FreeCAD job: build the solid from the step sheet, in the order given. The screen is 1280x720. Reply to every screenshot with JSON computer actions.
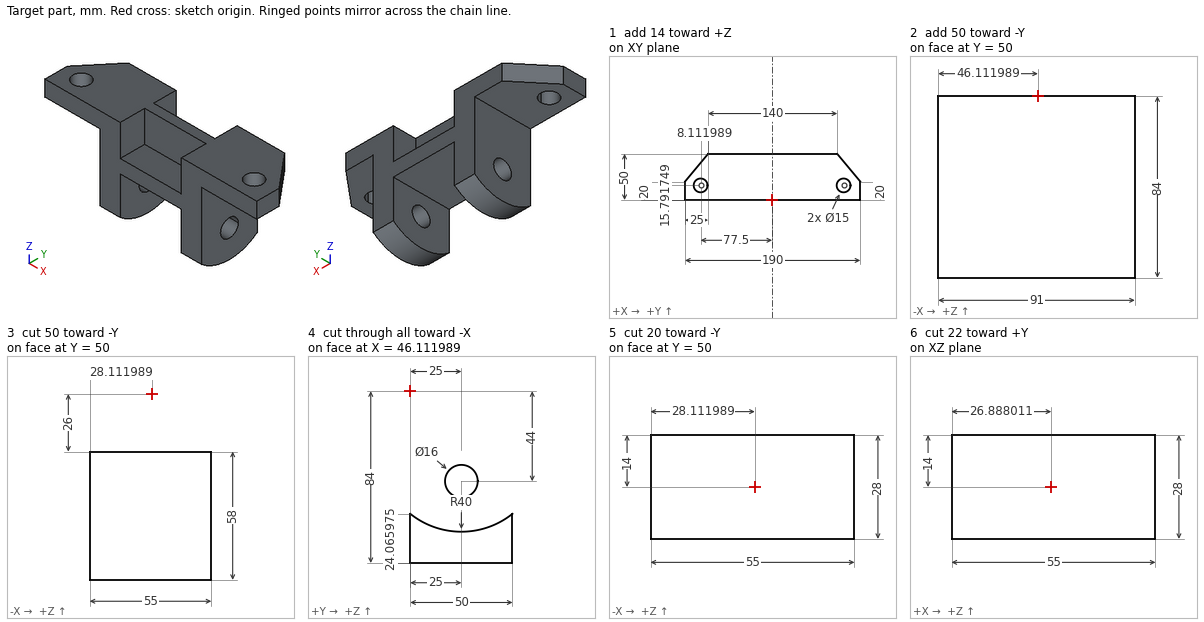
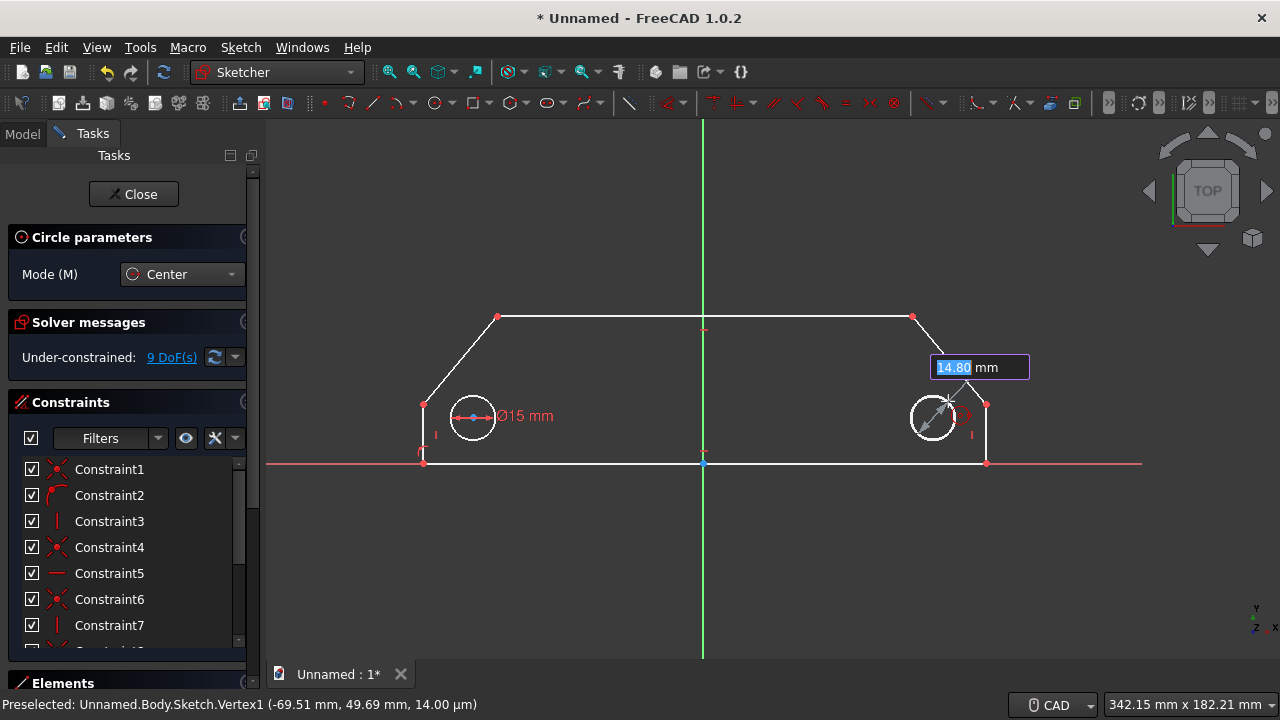
{"action": "type", "text": "15"}
{"action": "key", "text": "Return"}
{"action": "key", "text": "Escape"}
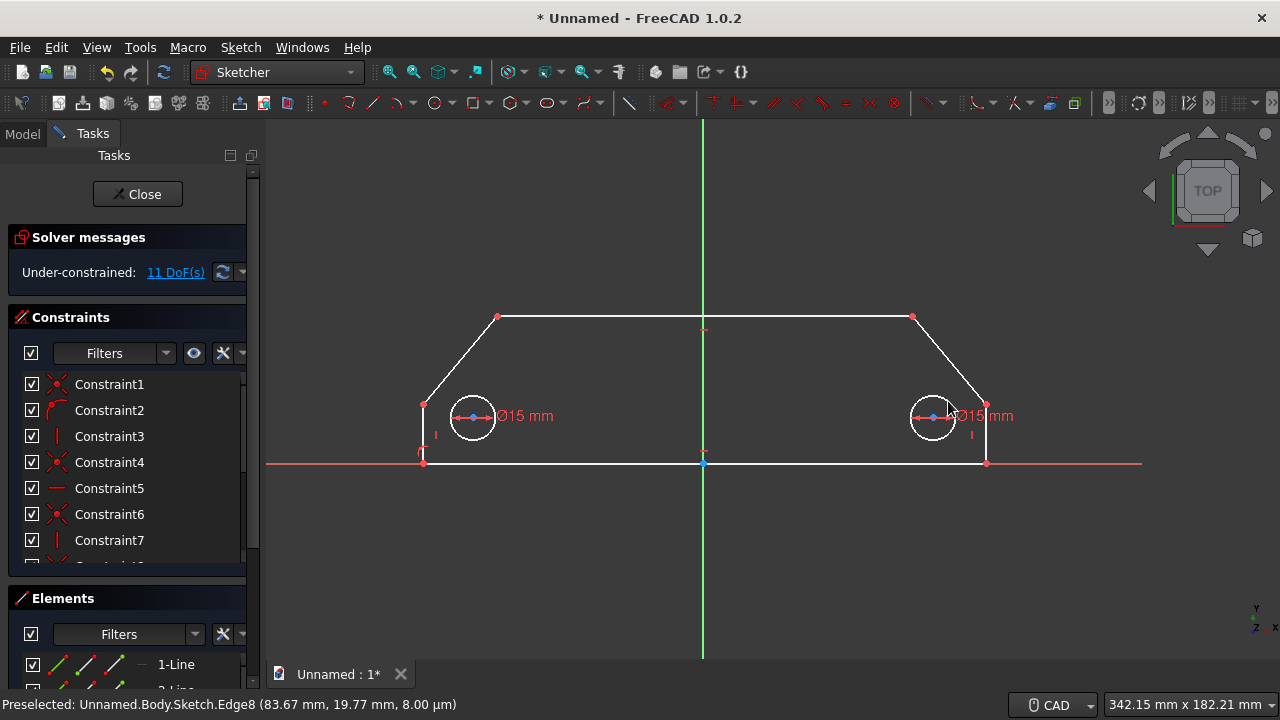
{"action": "left_click", "coordinate": [473, 418]}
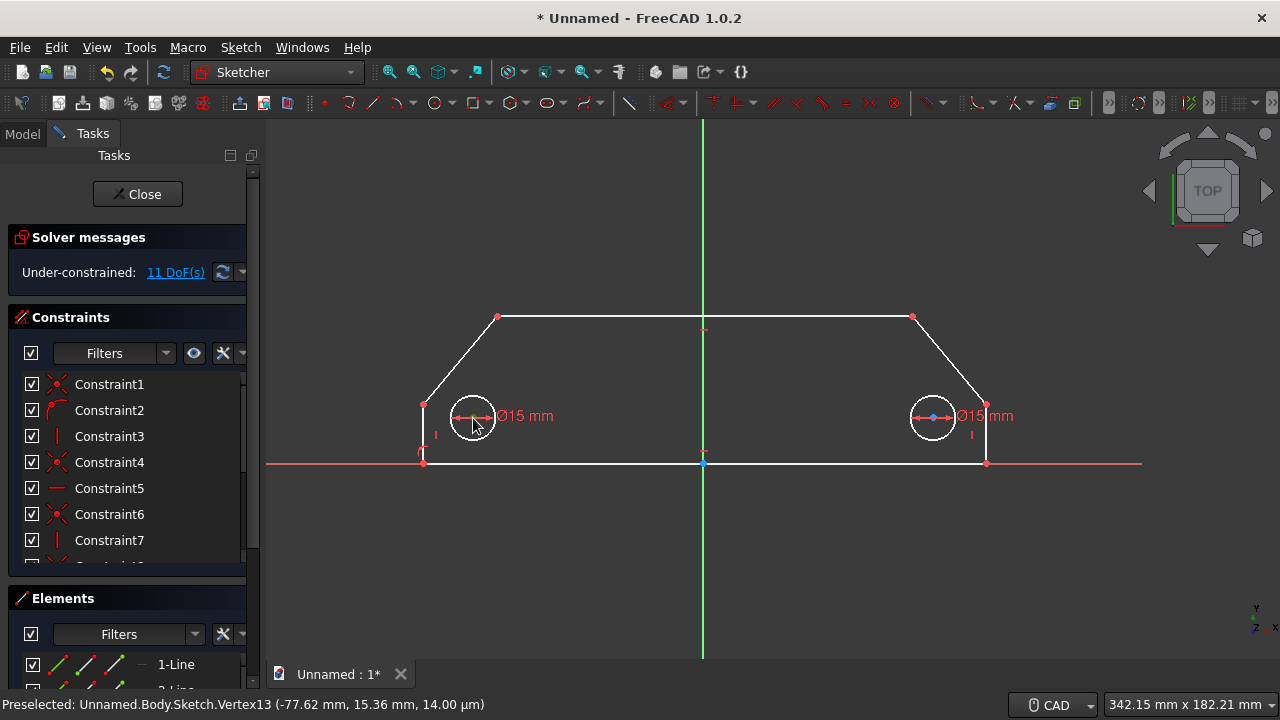
{"action": "left_click", "coordinate": [933, 418]}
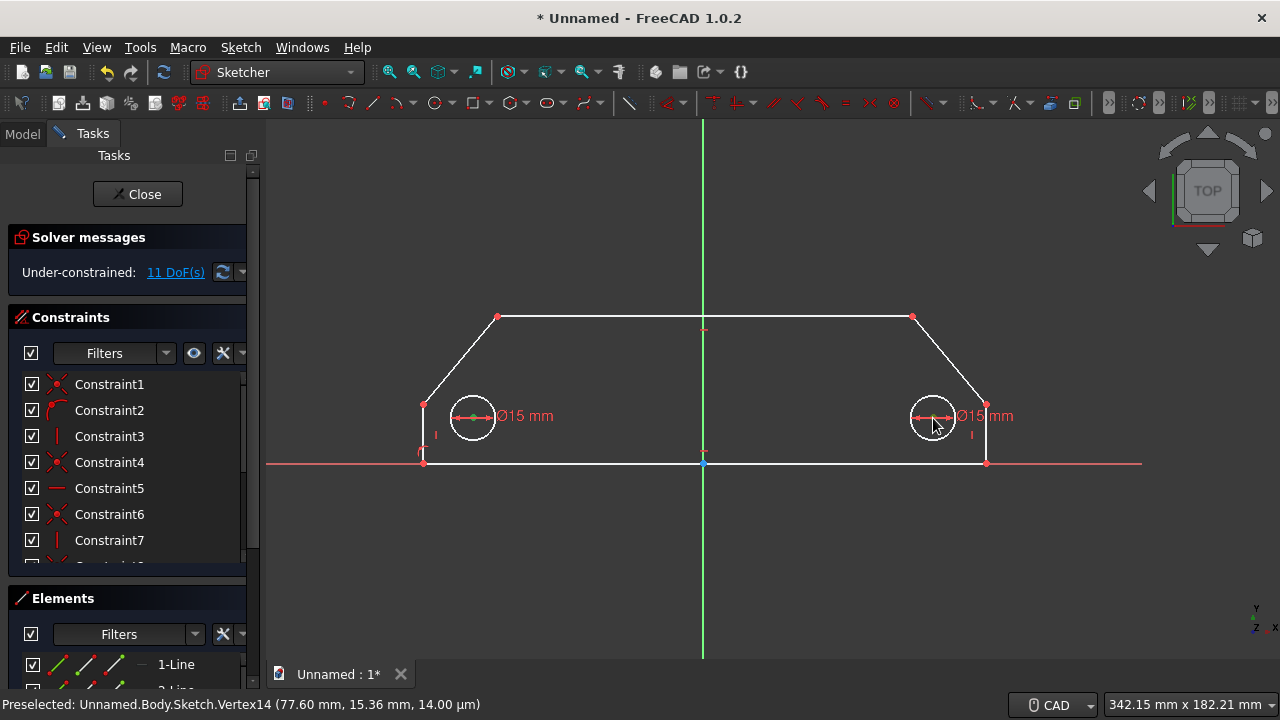
{"action": "left_click", "coordinate": [703, 596]}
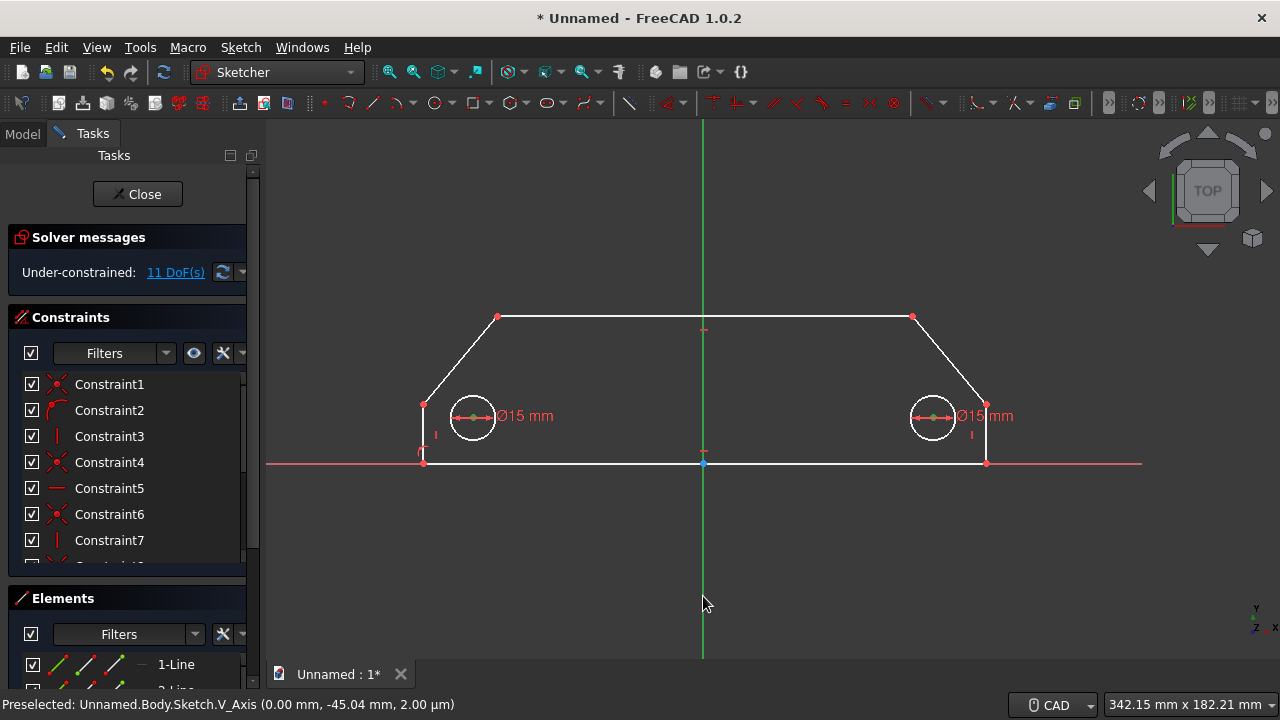
{"action": "left_click", "coordinate": [870, 104]}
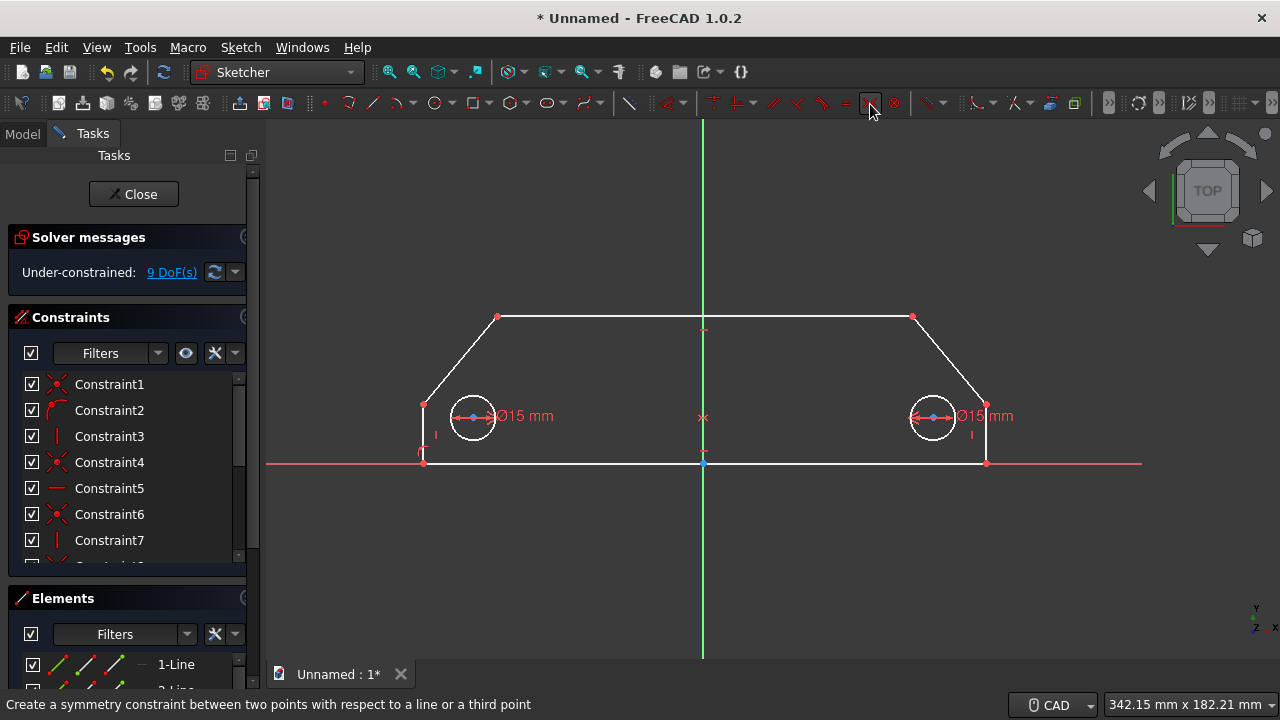
{"action": "left_click", "coordinate": [668, 104]}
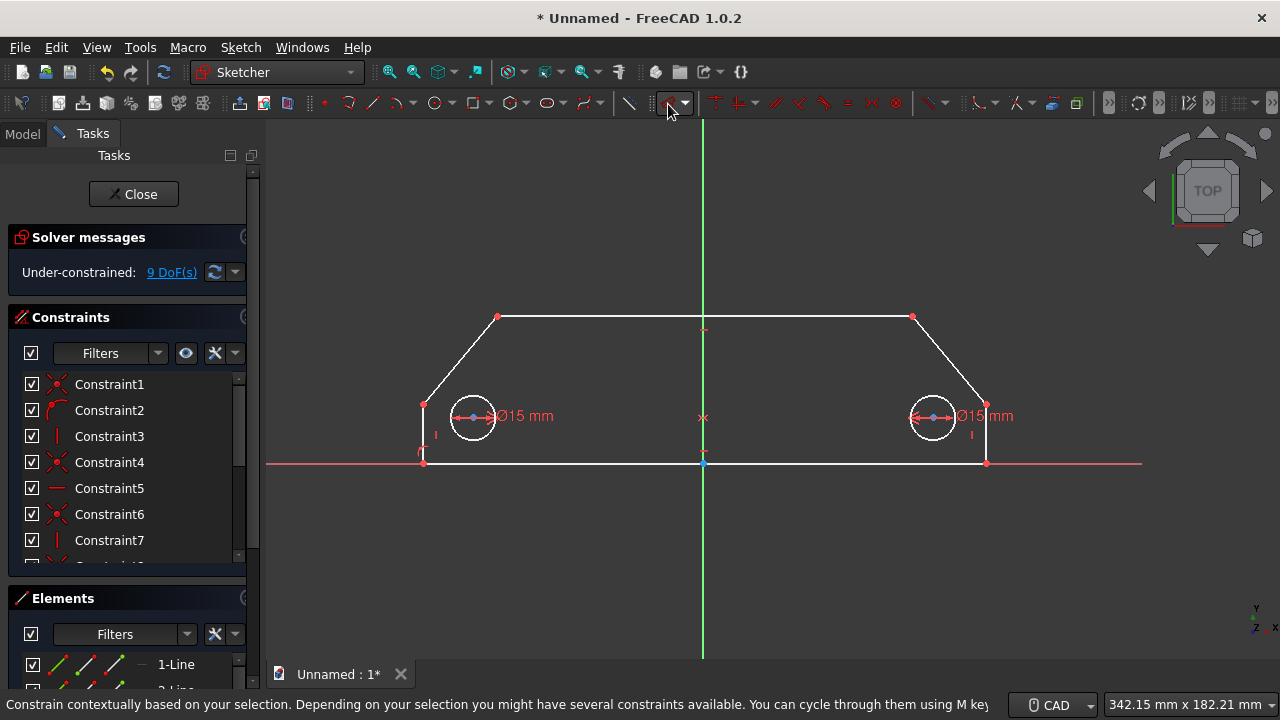
{"action": "left_click", "coordinate": [423, 423]}
{"action": "left_click", "coordinate": [389, 434]}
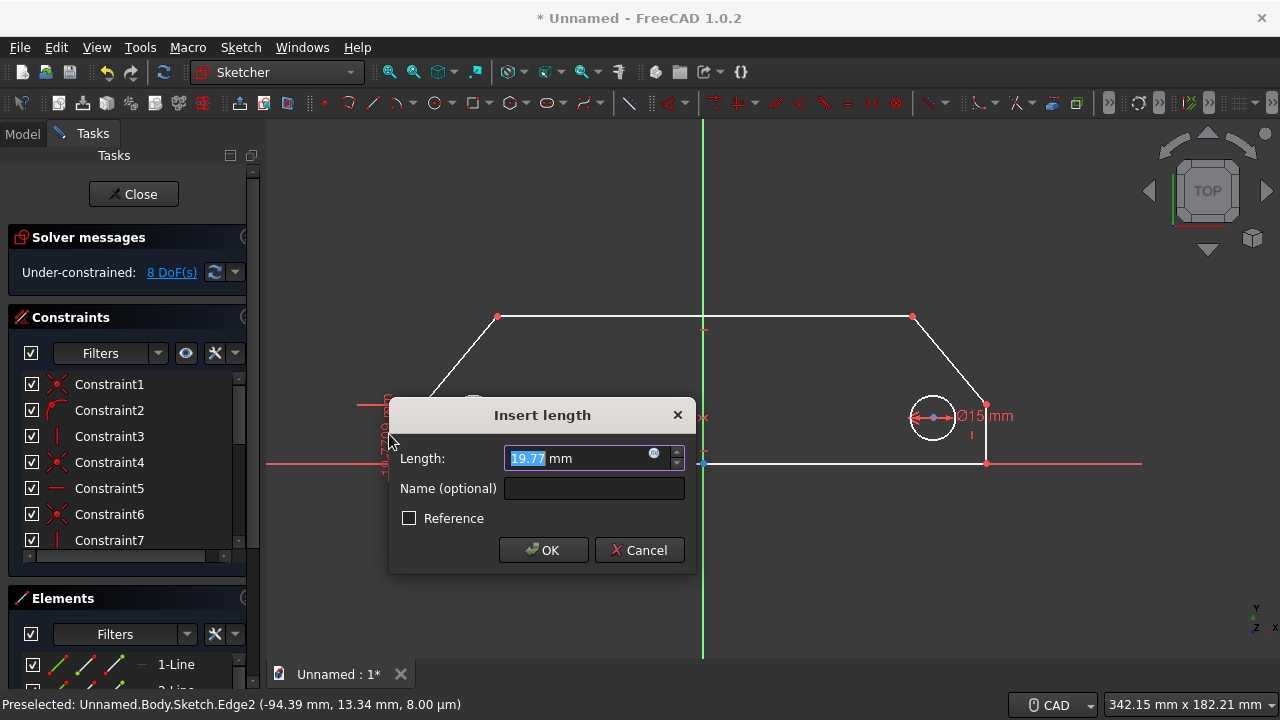
{"action": "type", "text": "20"}
{"action": "key", "text": "Return"}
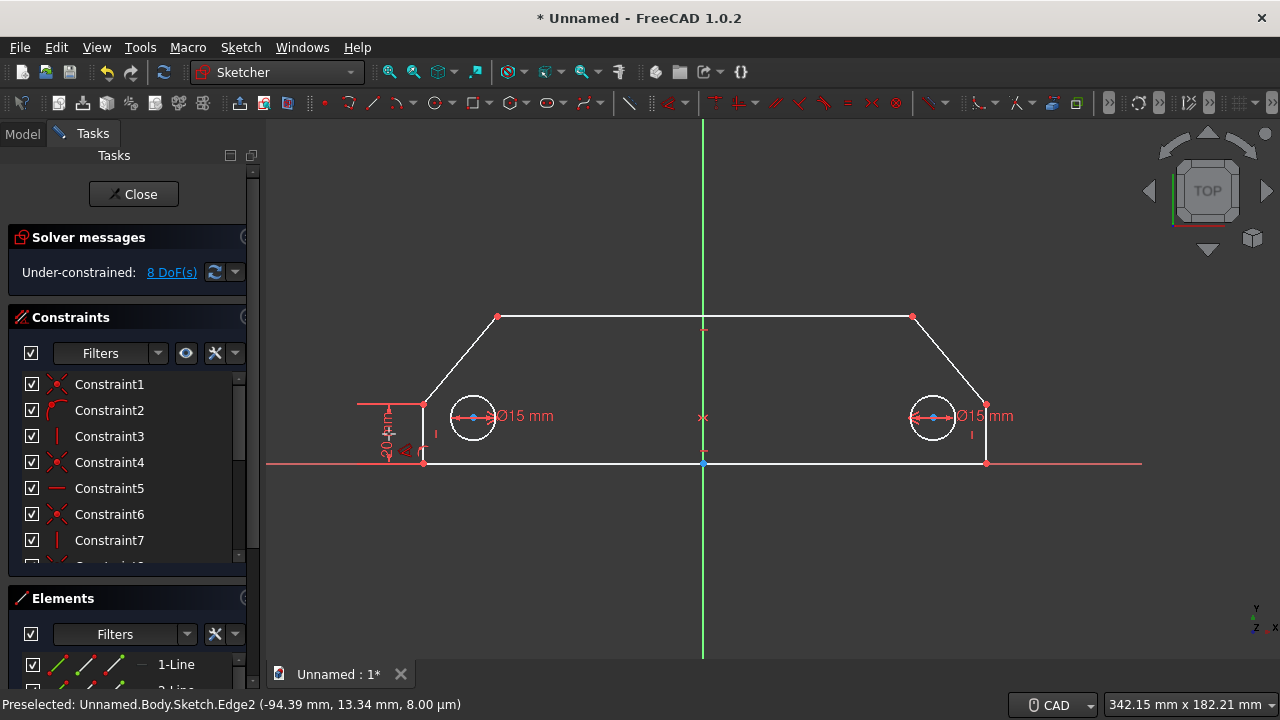
{"action": "left_click", "coordinate": [986, 446]}
{"action": "left_click", "coordinate": [1020, 434]}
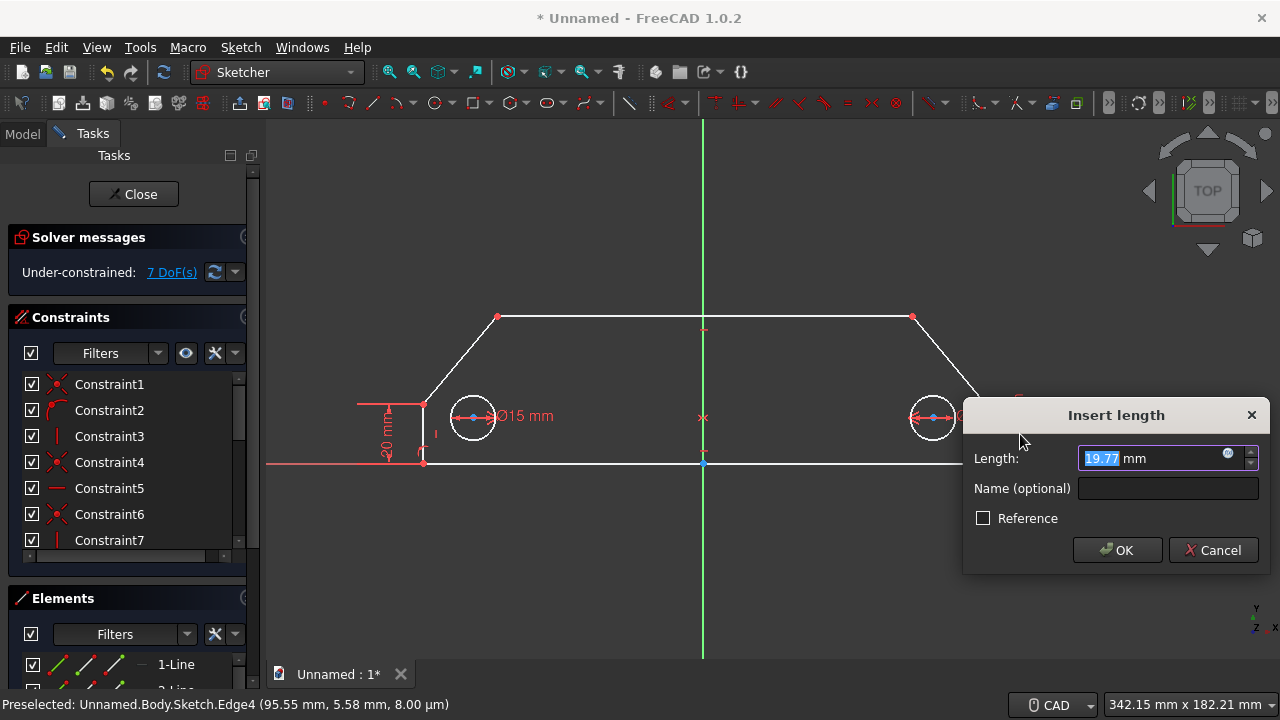
{"action": "type", "text": "20"}
{"action": "key", "text": "Return"}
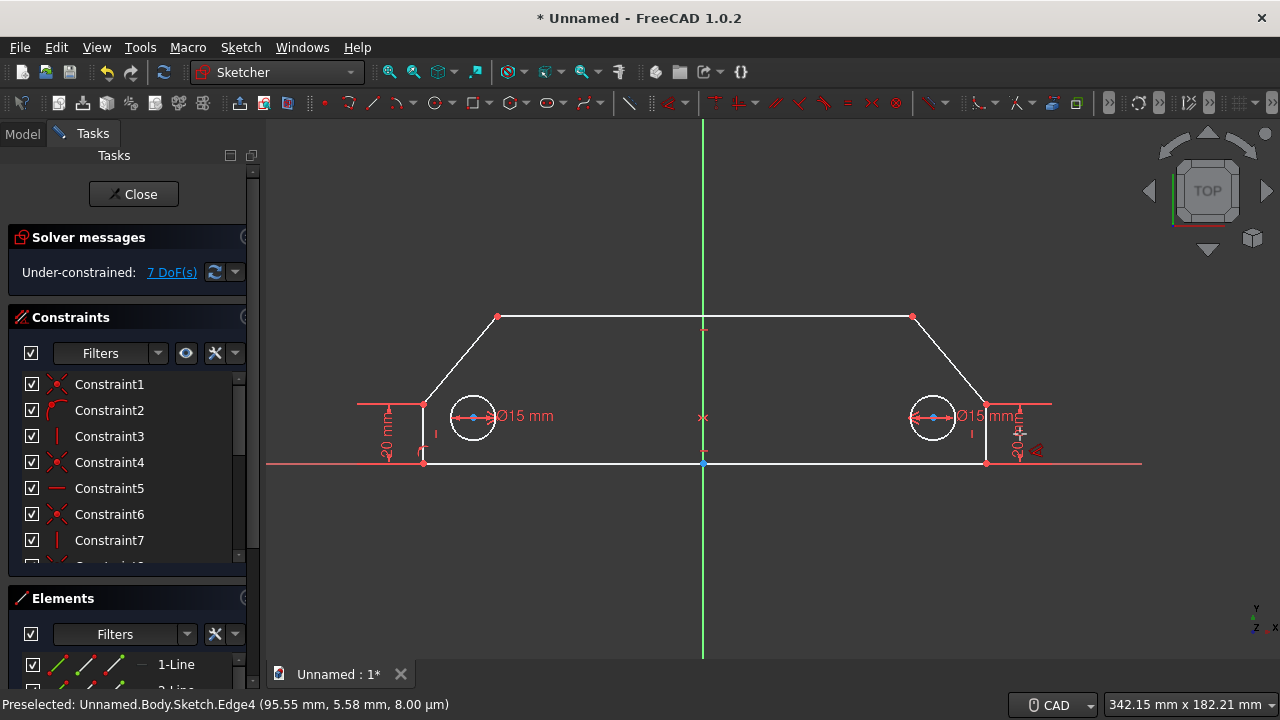
{"action": "left_click", "coordinate": [592, 464]}
{"action": "left_click", "coordinate": [575, 498]}